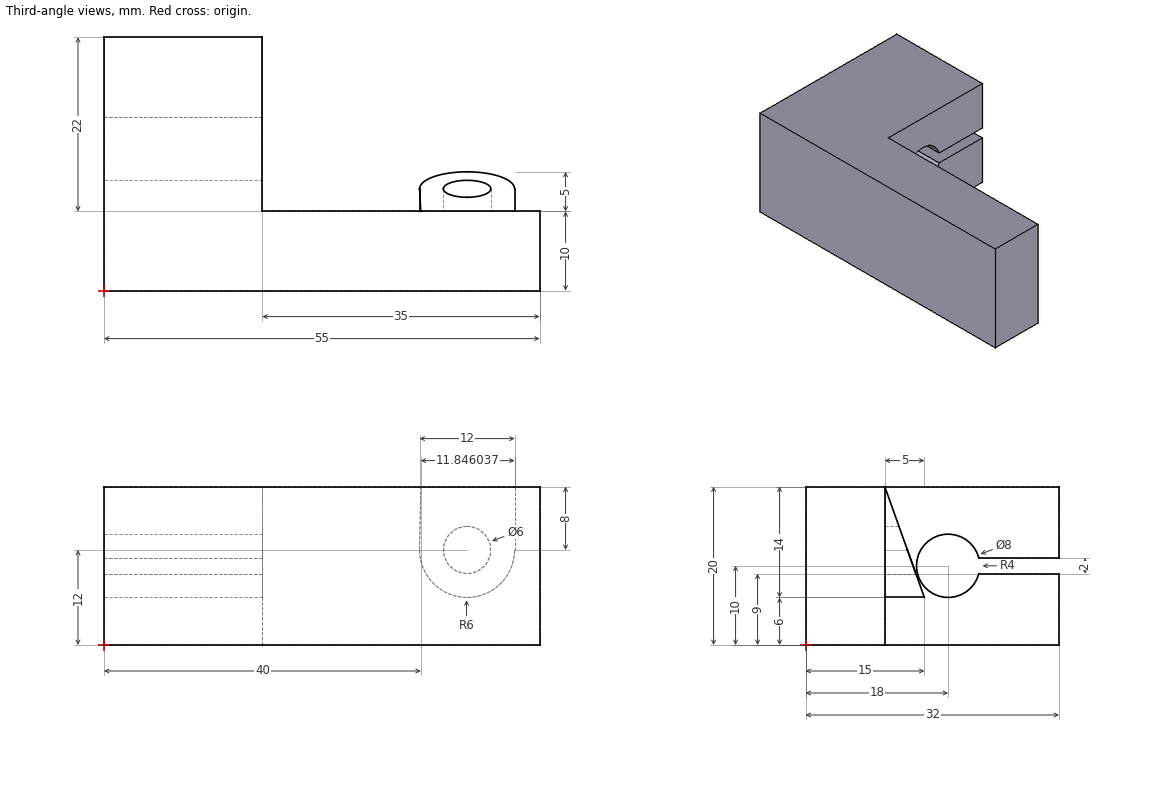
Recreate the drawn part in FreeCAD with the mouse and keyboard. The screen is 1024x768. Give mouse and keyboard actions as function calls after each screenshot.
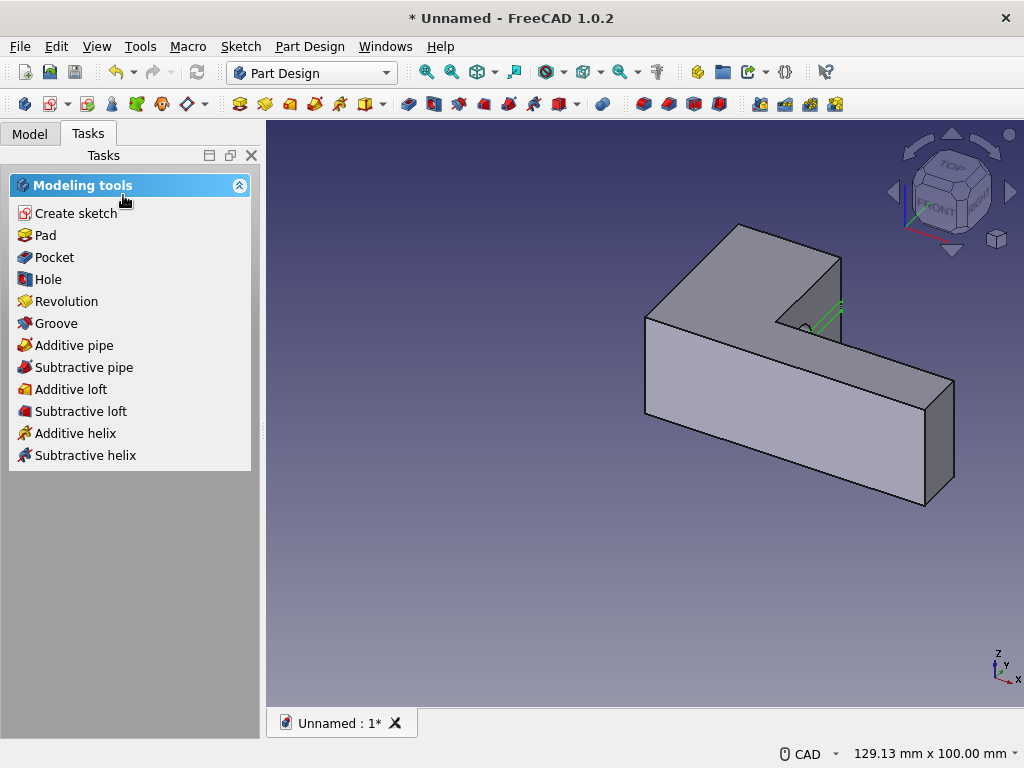
click(409, 104)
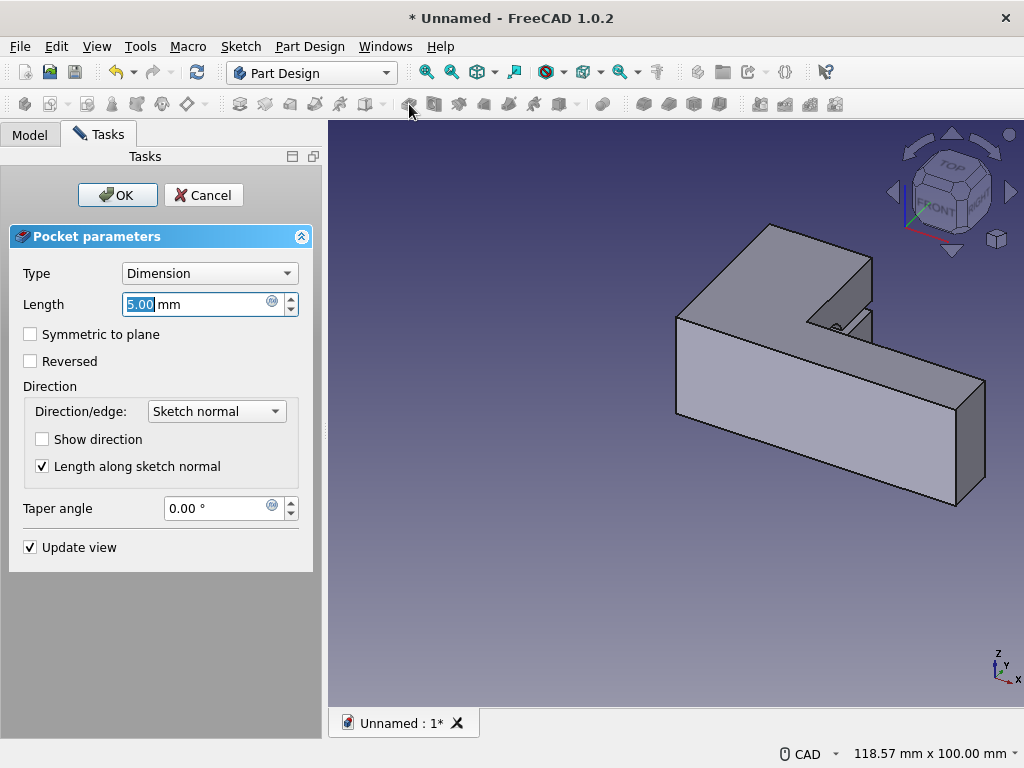
click(210, 274)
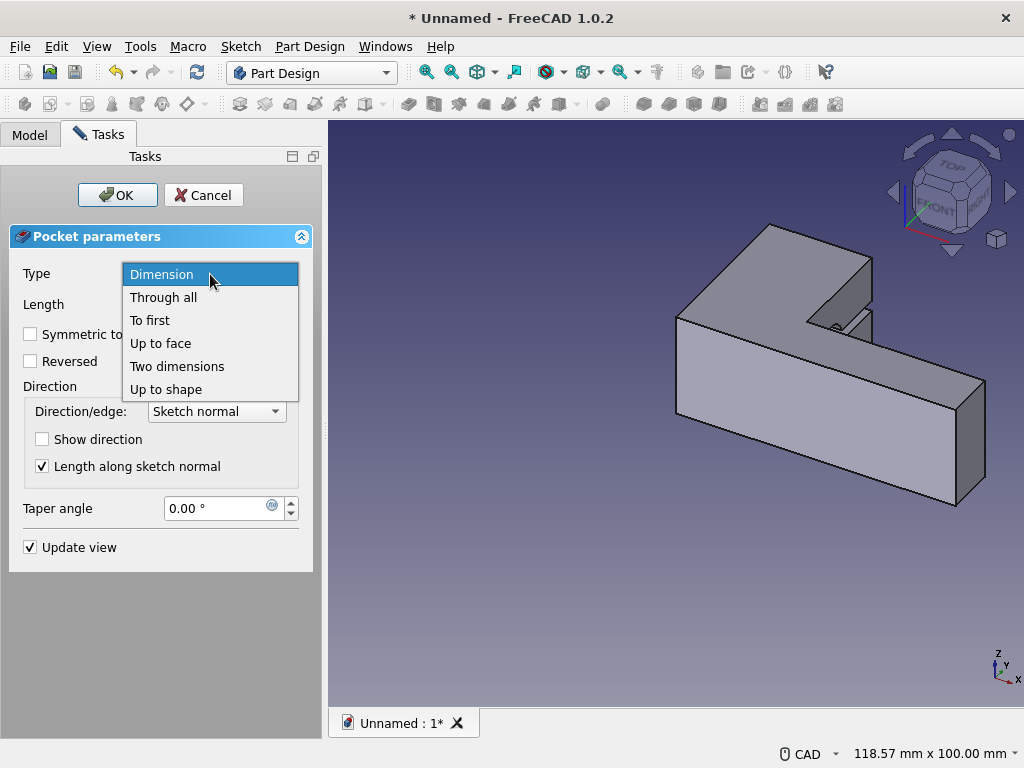
click(208, 298)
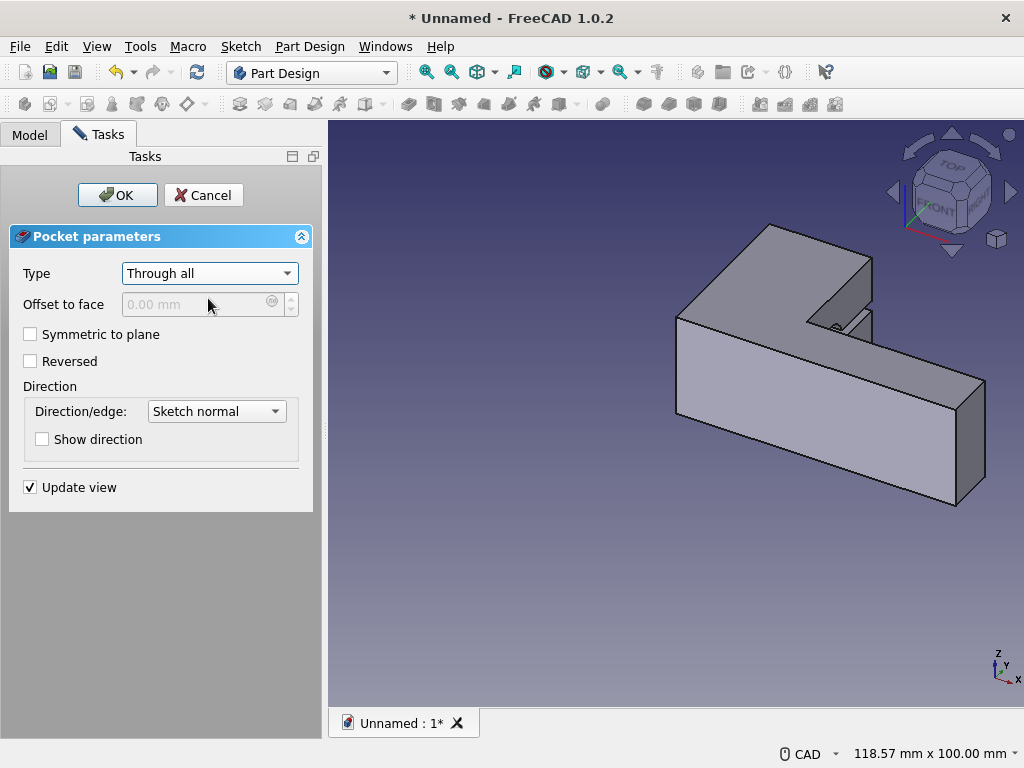
click(118, 195)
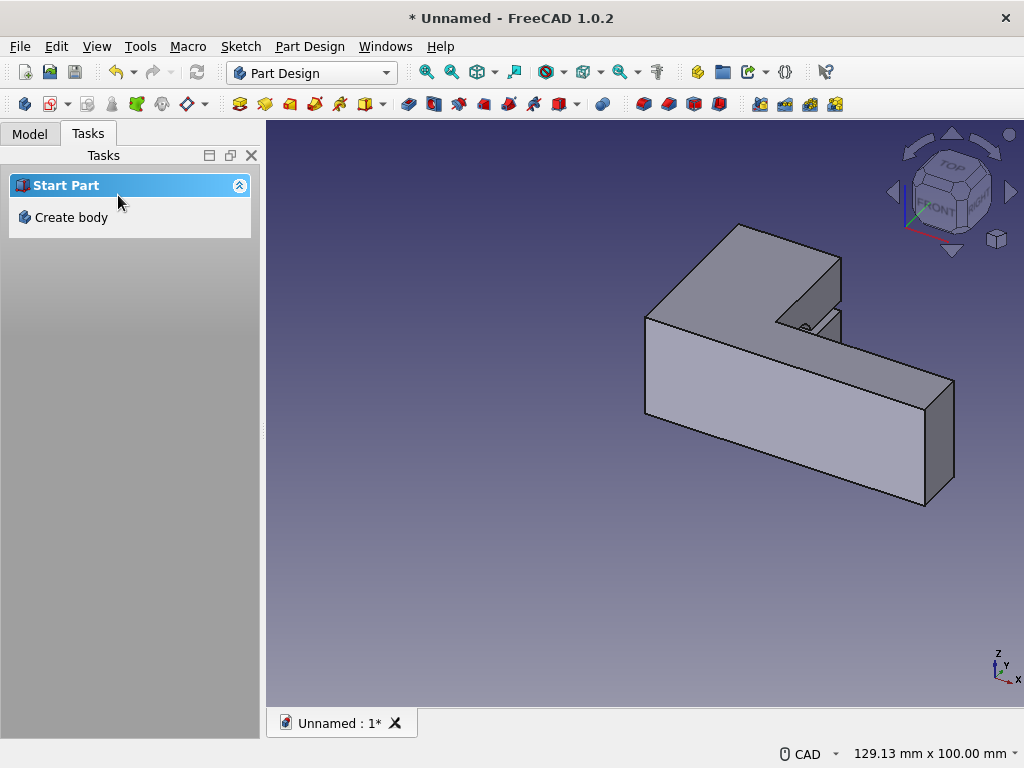
key(4)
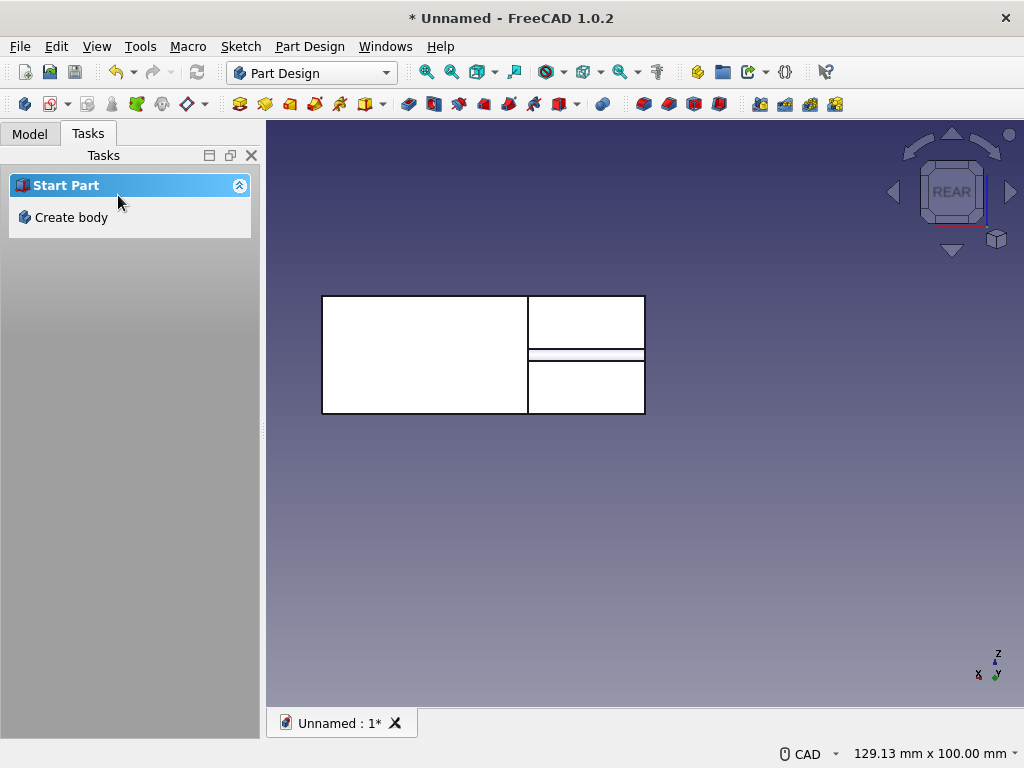
key(v)
key(f)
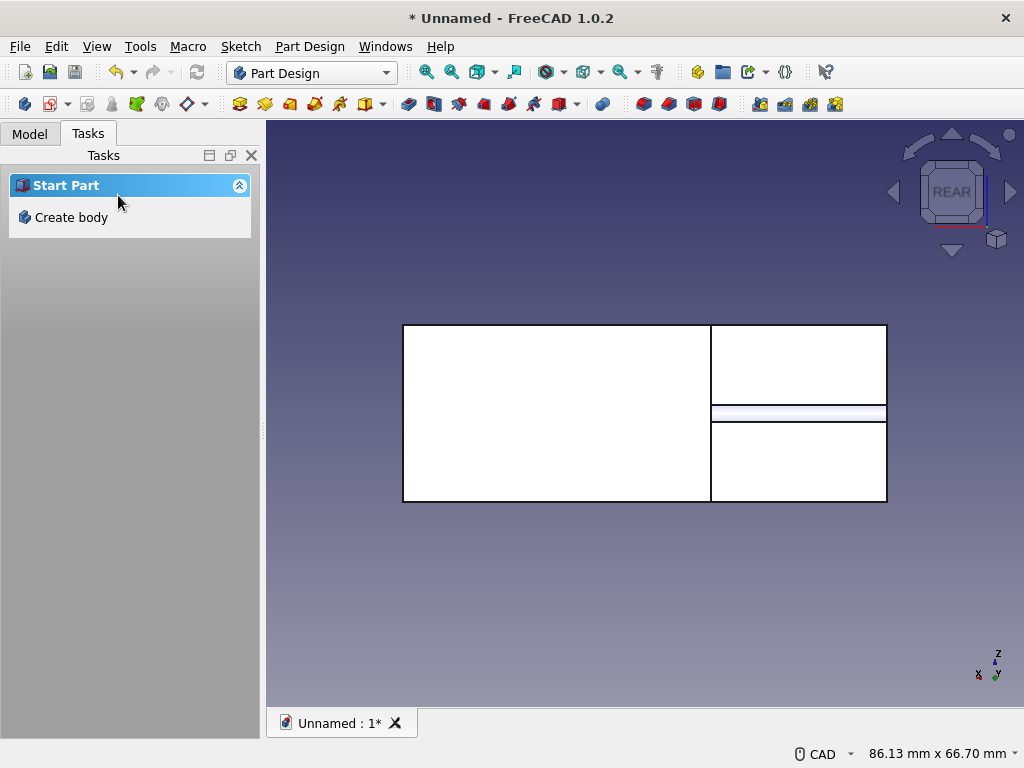
click(513, 413)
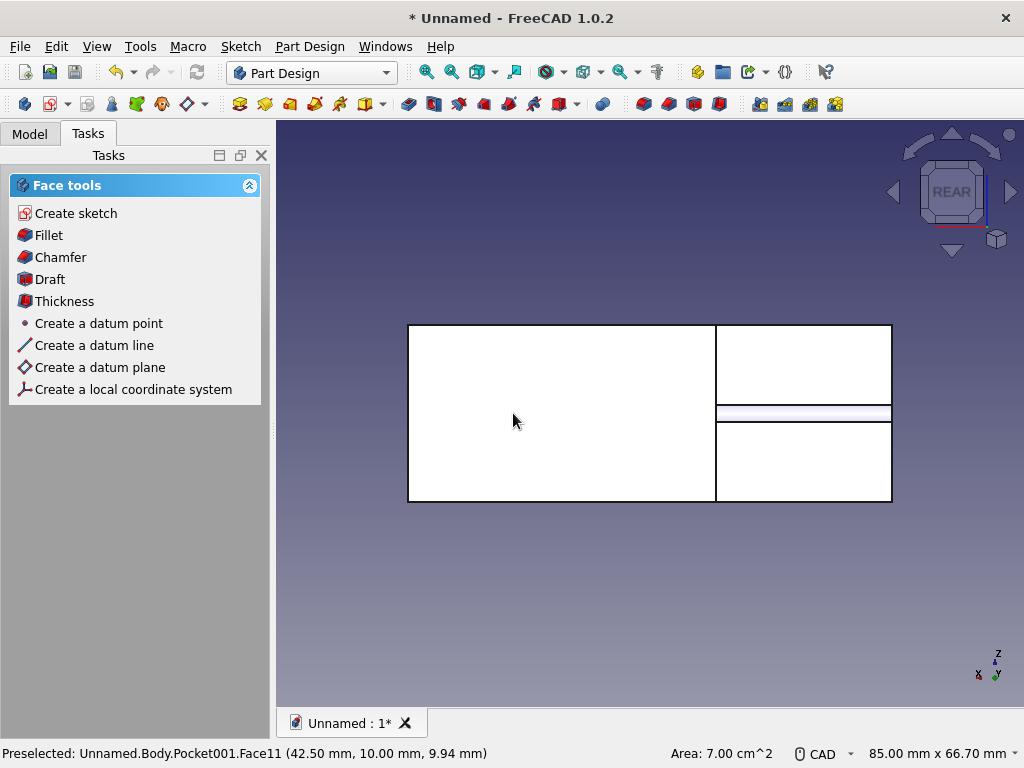
click(50, 104)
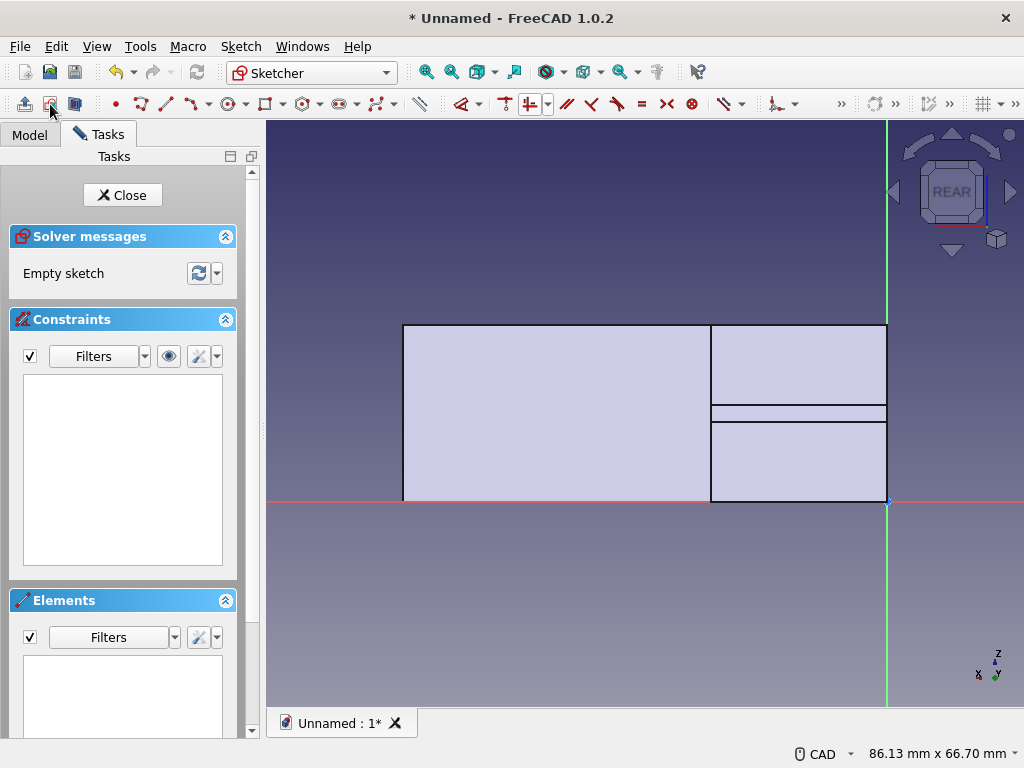
click(75, 104)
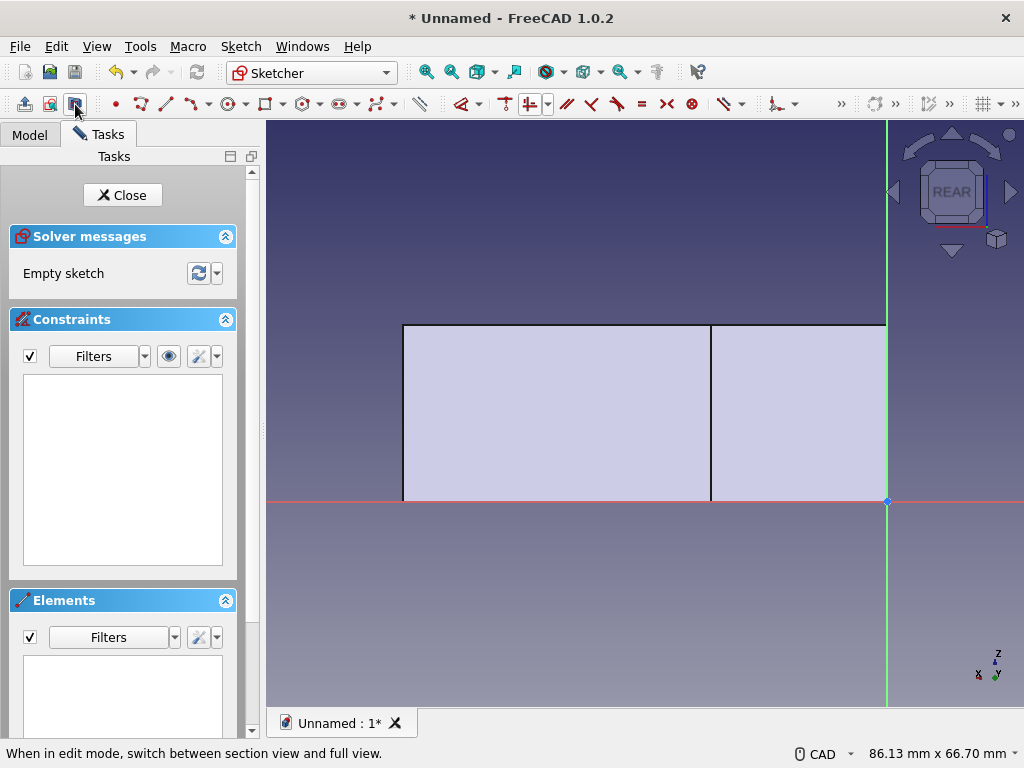
scroll(443, 376, up, 6)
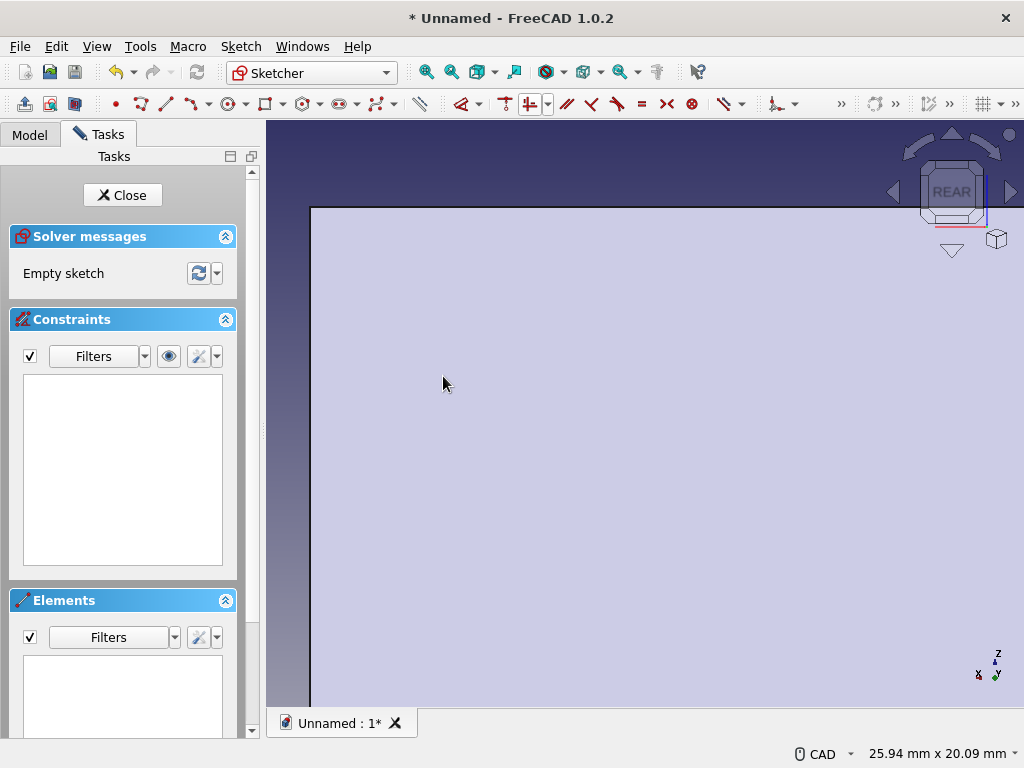
key(g)
key(m)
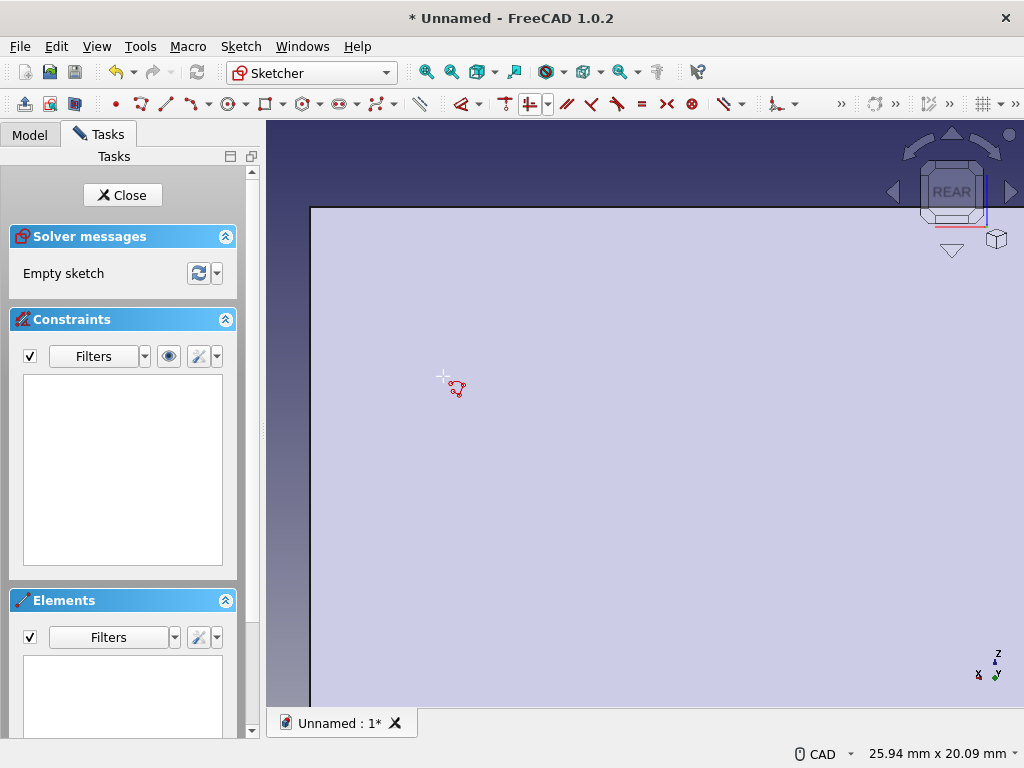
click(752, 438)
click(740, 207)
click(402, 207)
click(402, 441)
right_click(402, 441)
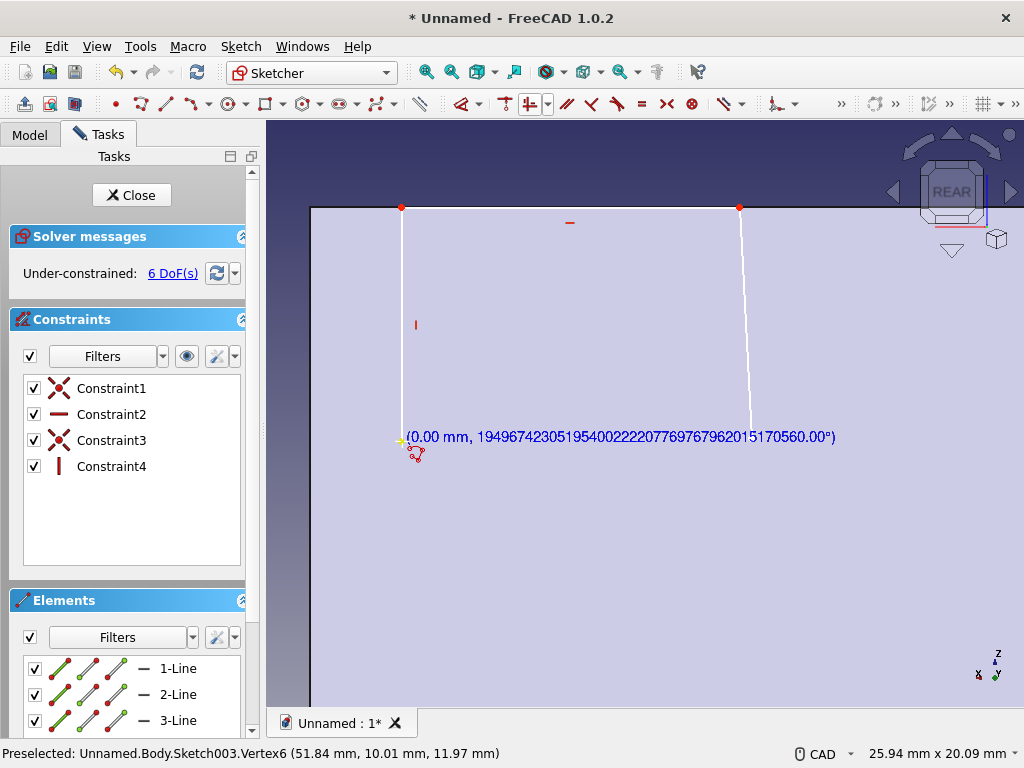
key(g)
key(3)
key(a)